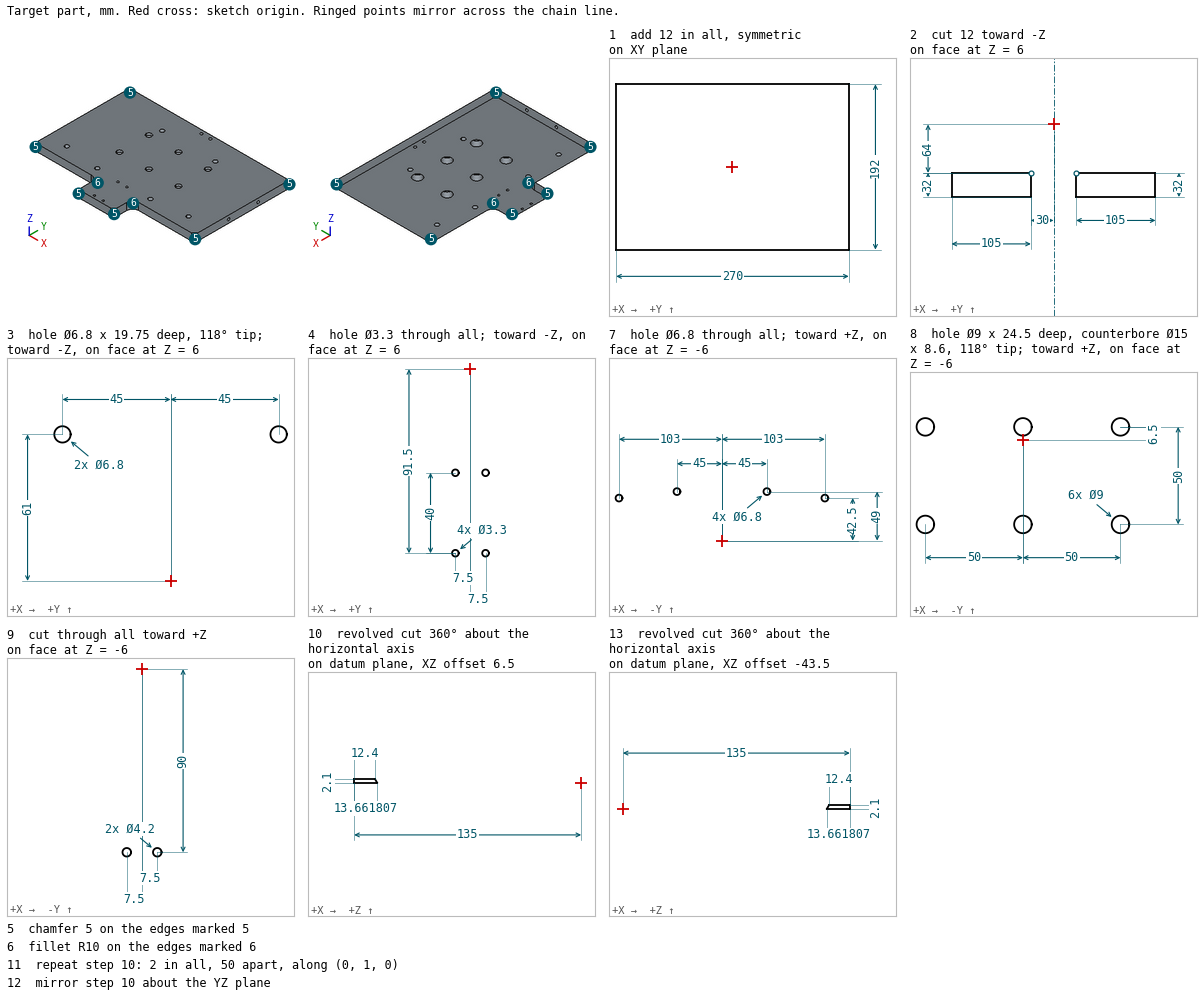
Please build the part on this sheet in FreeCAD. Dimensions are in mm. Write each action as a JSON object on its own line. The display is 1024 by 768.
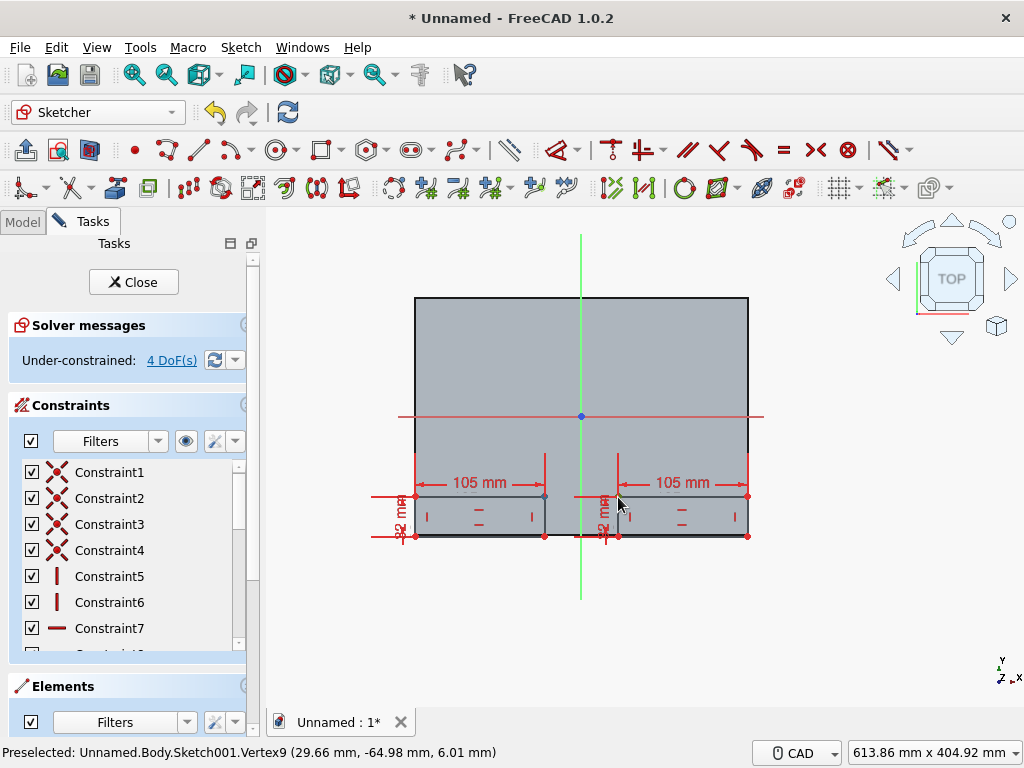
{"action": "left_click", "coordinate": [581, 584]}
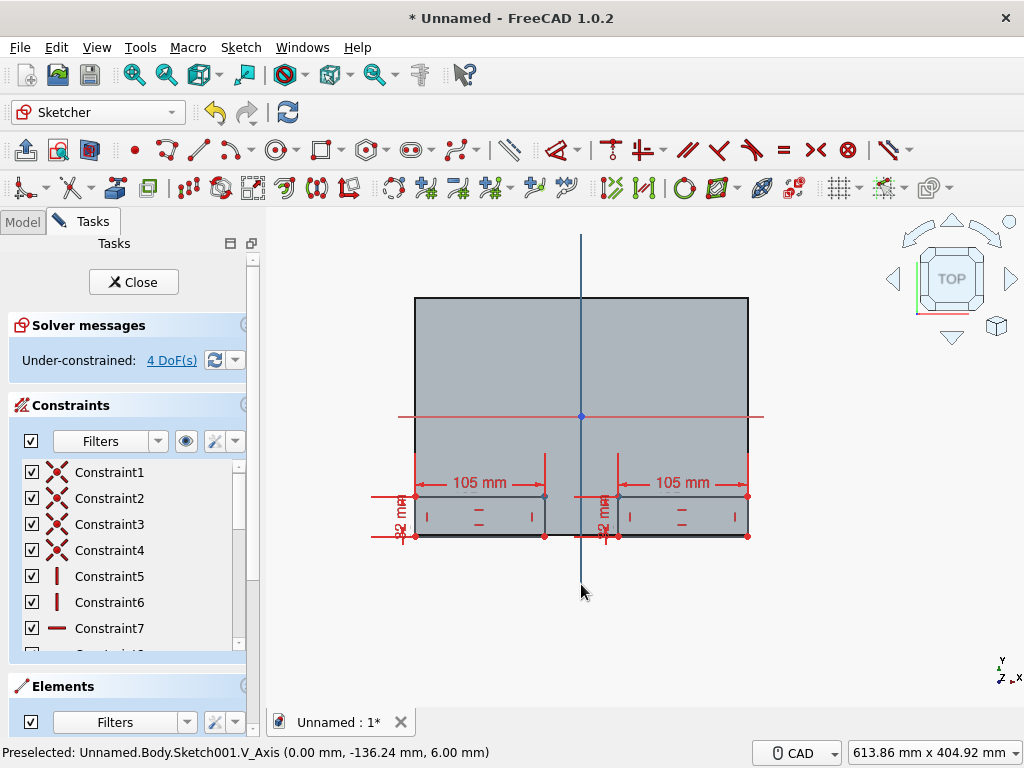
{"action": "key", "text": "s"}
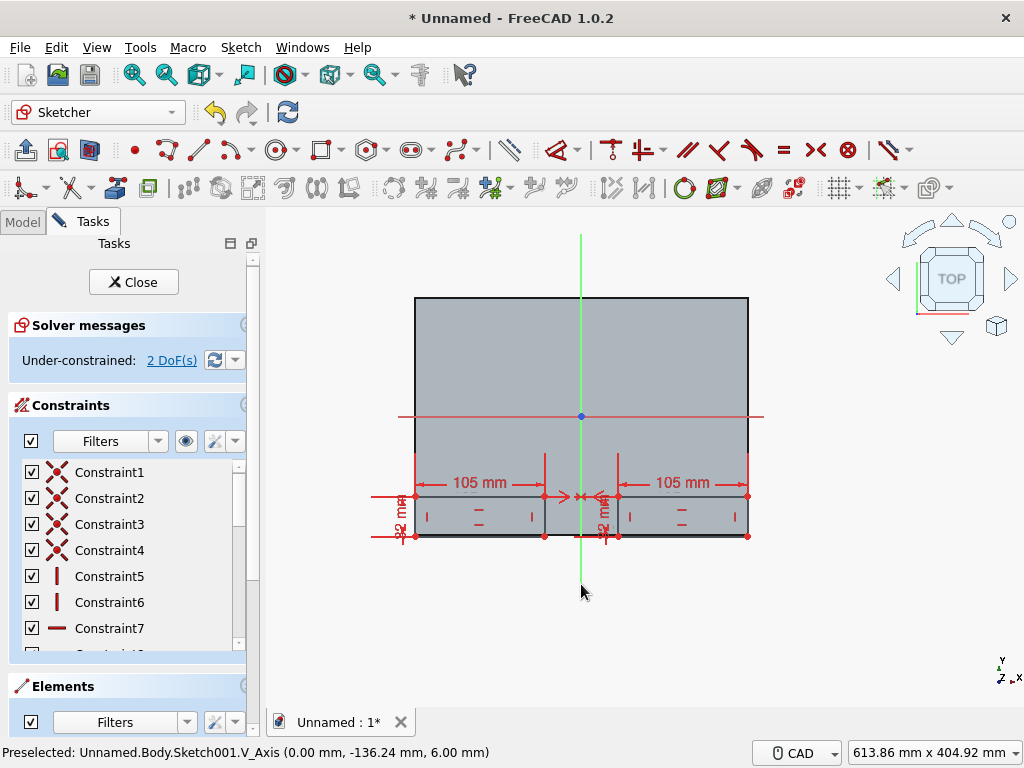
{"action": "key", "text": "d"}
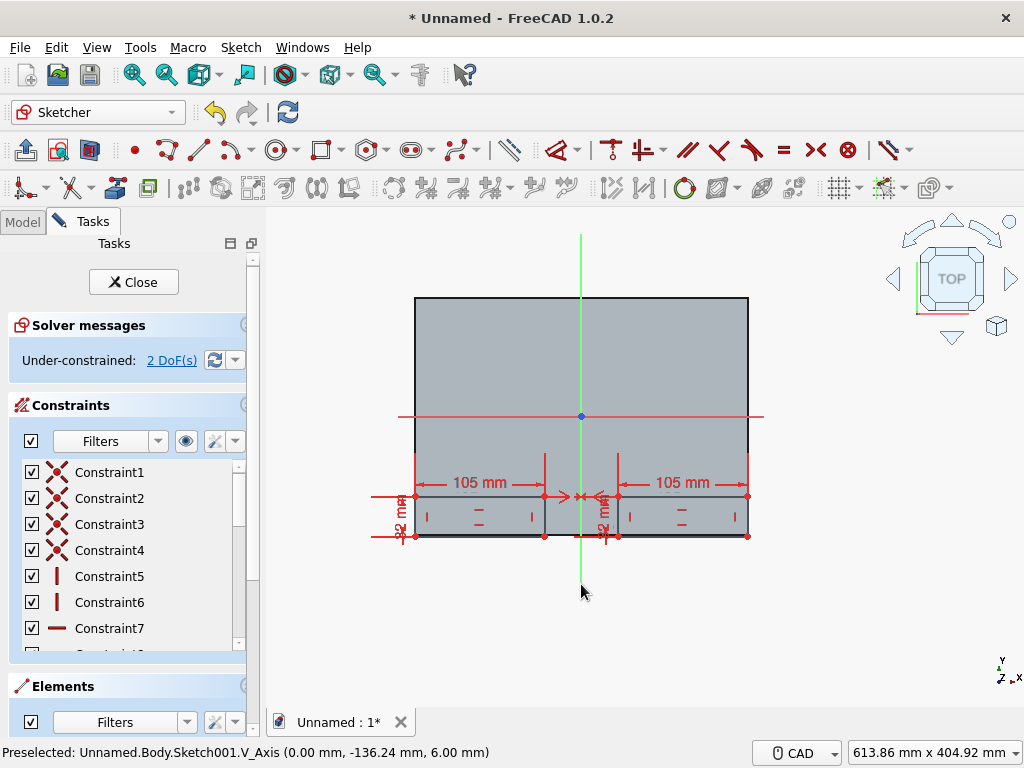
{"action": "left_click", "coordinate": [415, 497]}
{"action": "left_click", "coordinate": [381, 457]}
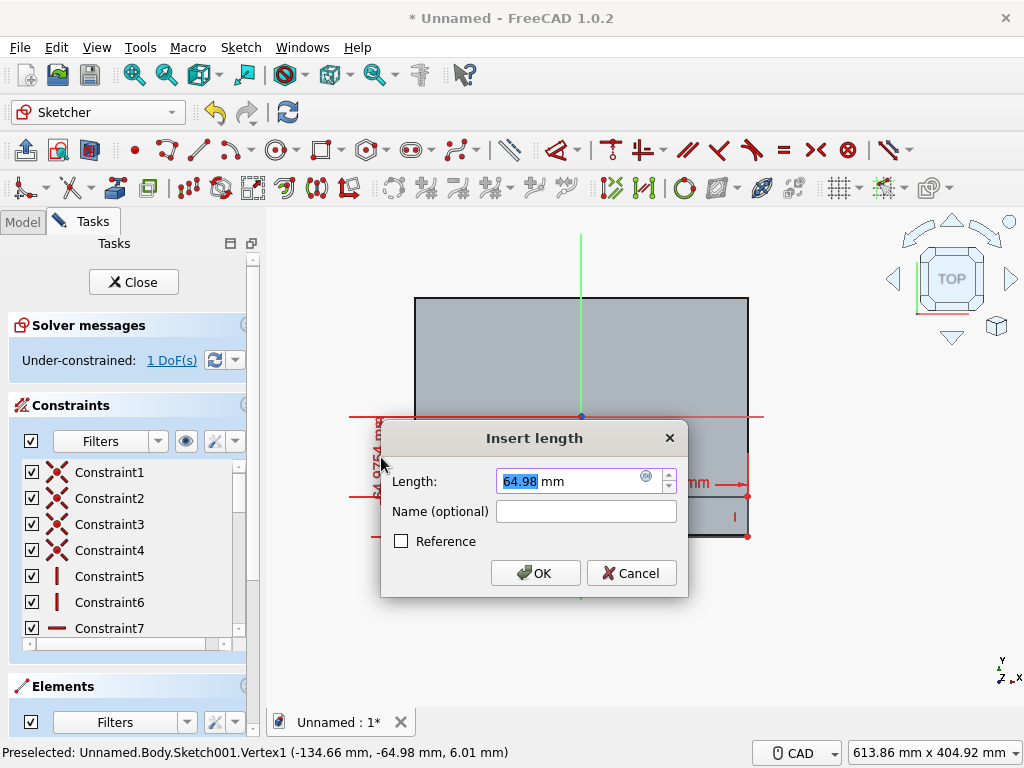
{"action": "type", "text": "64"}
{"action": "key", "text": "Return"}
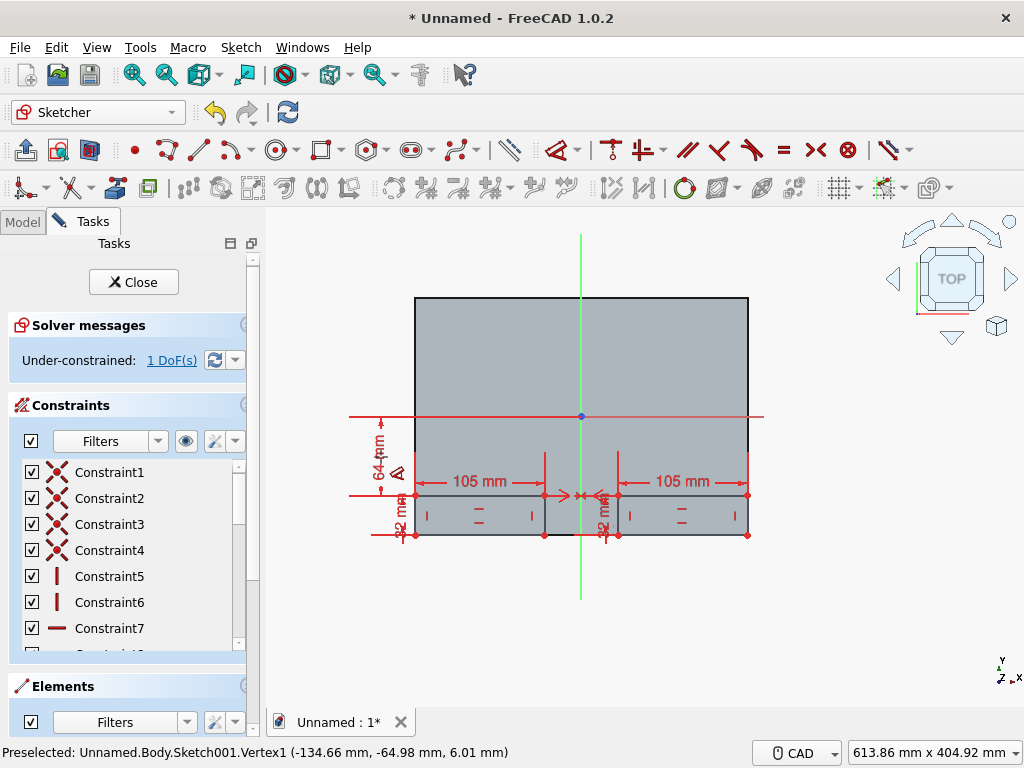
{"action": "left_click", "coordinate": [545, 535]}
{"action": "left_click", "coordinate": [563, 569]}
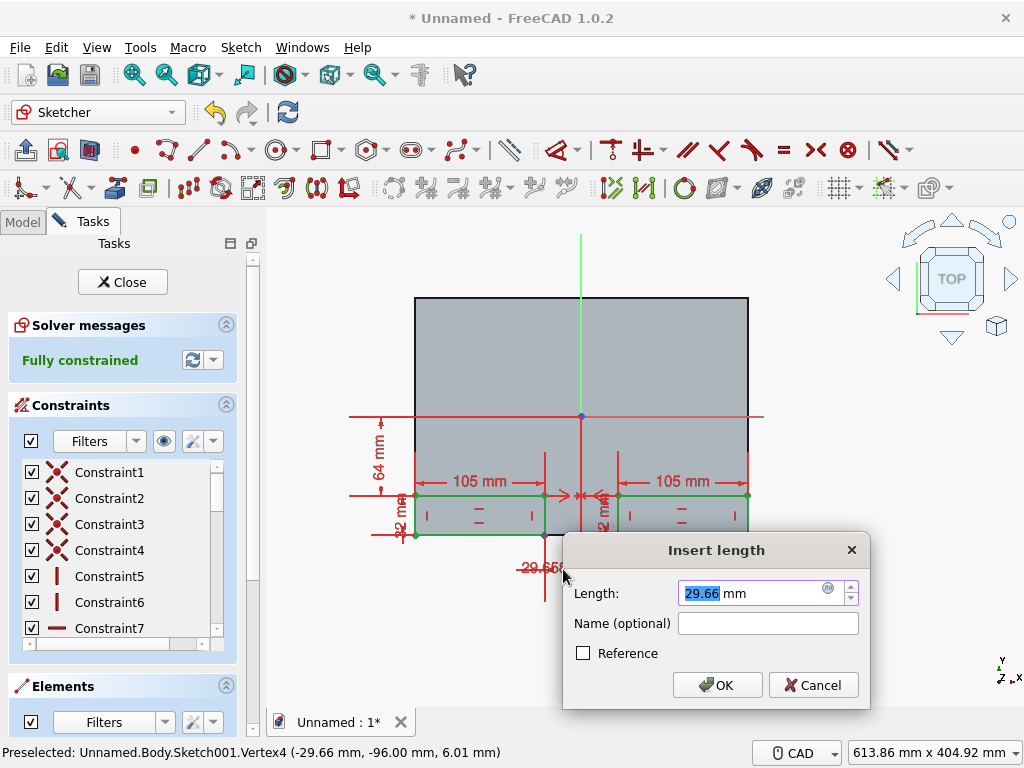
{"action": "type", "text": "30"}
{"action": "key", "text": "Return"}
{"action": "key", "text": "Escape"}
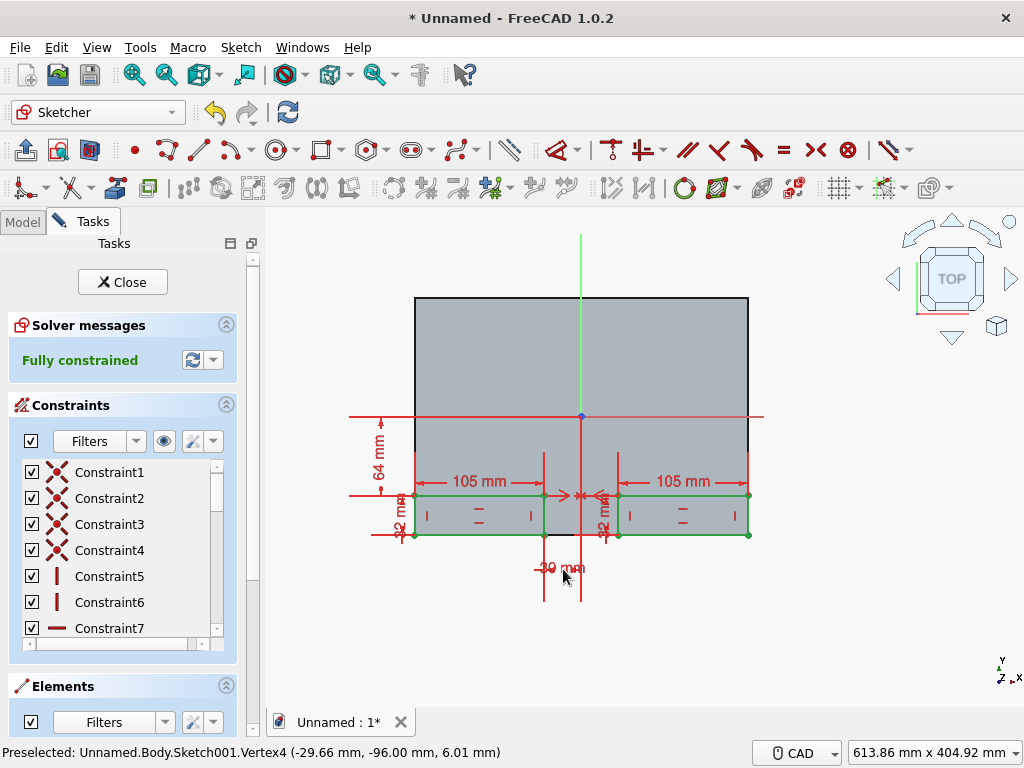
{"action": "left_click", "coordinate": [123, 282]}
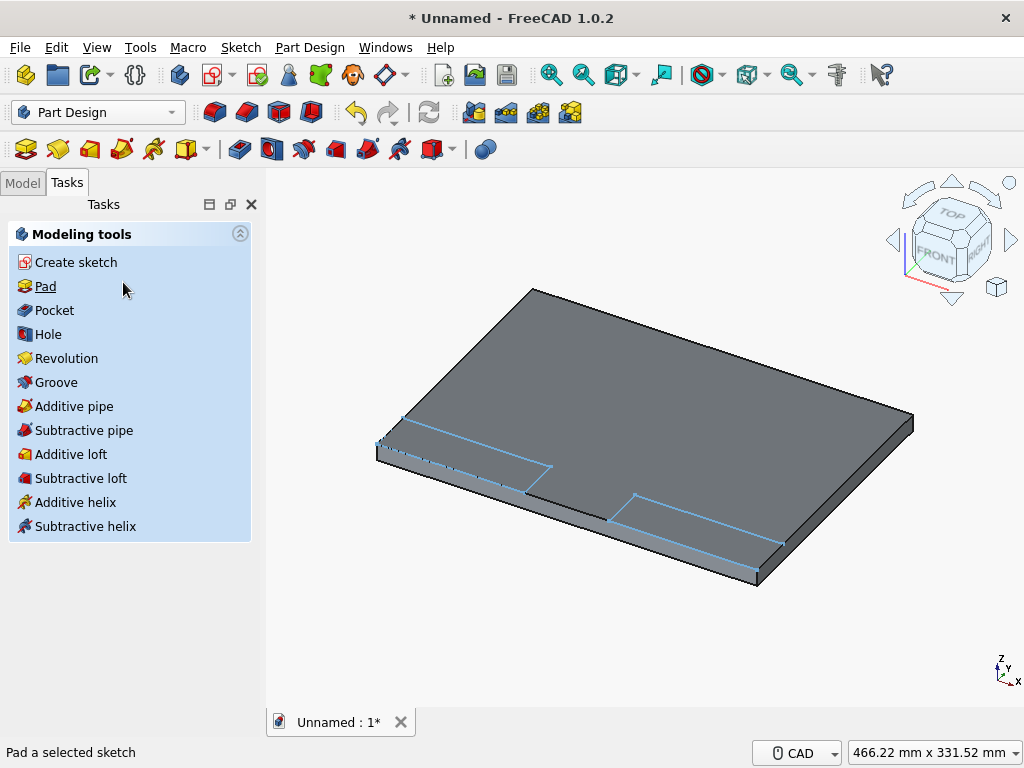
{"action": "left_click", "coordinate": [240, 150]}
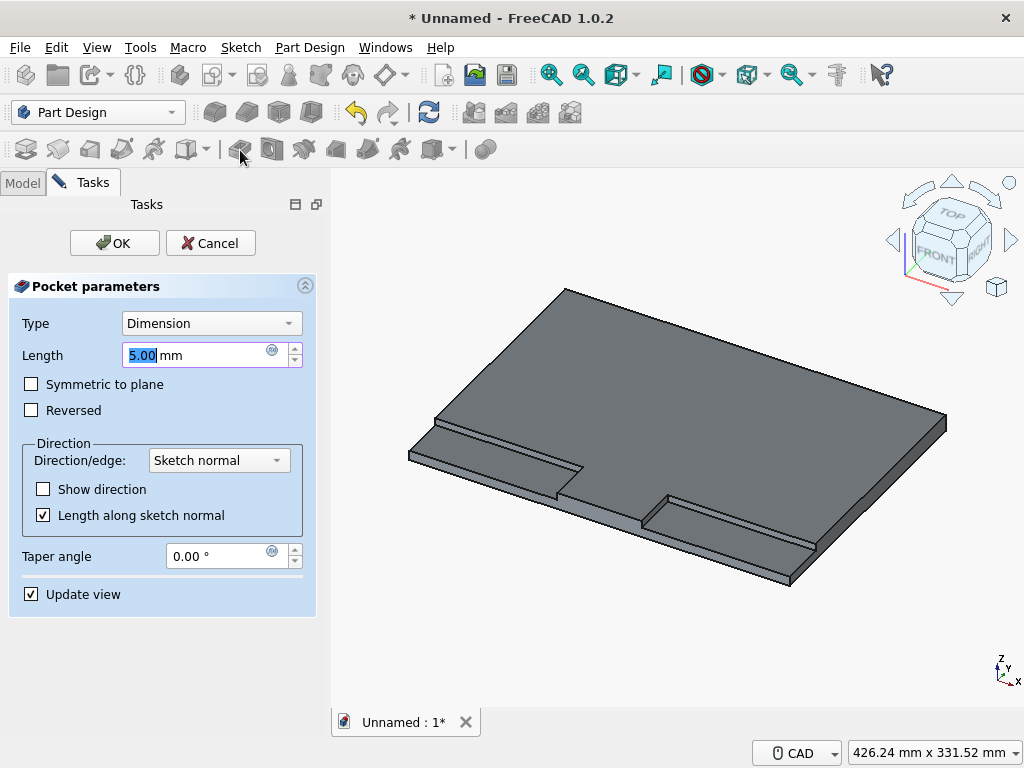
{"action": "type", "text": "12"}
{"action": "key", "text": "Tab"}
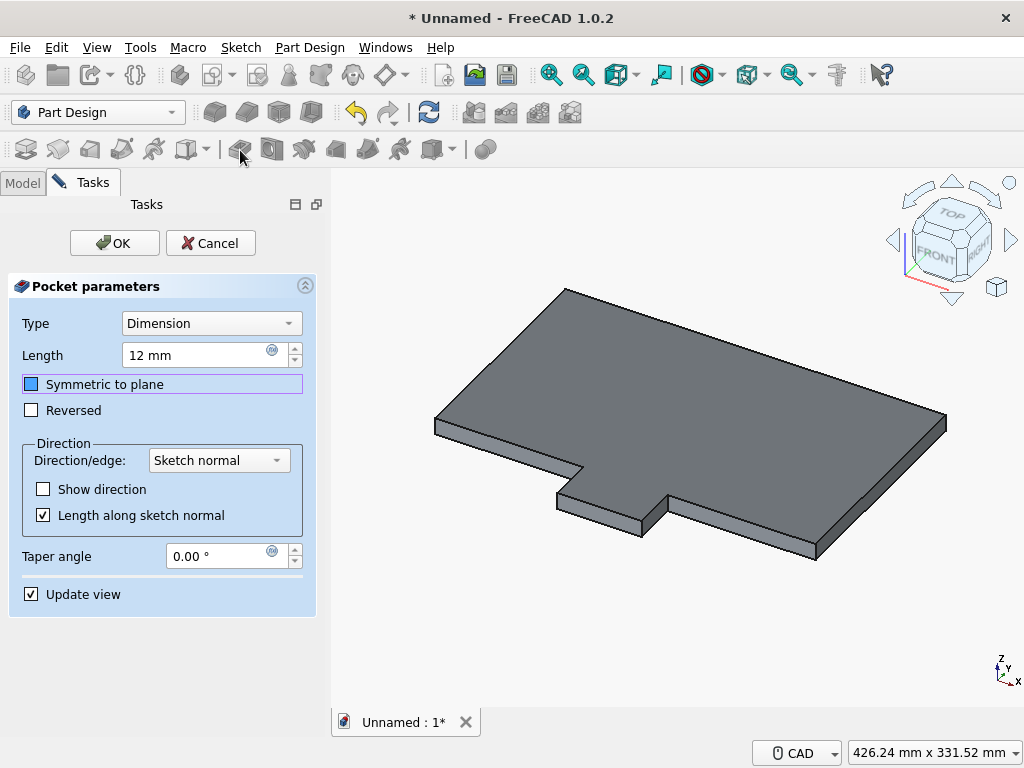
{"action": "left_click", "coordinate": [115, 243]}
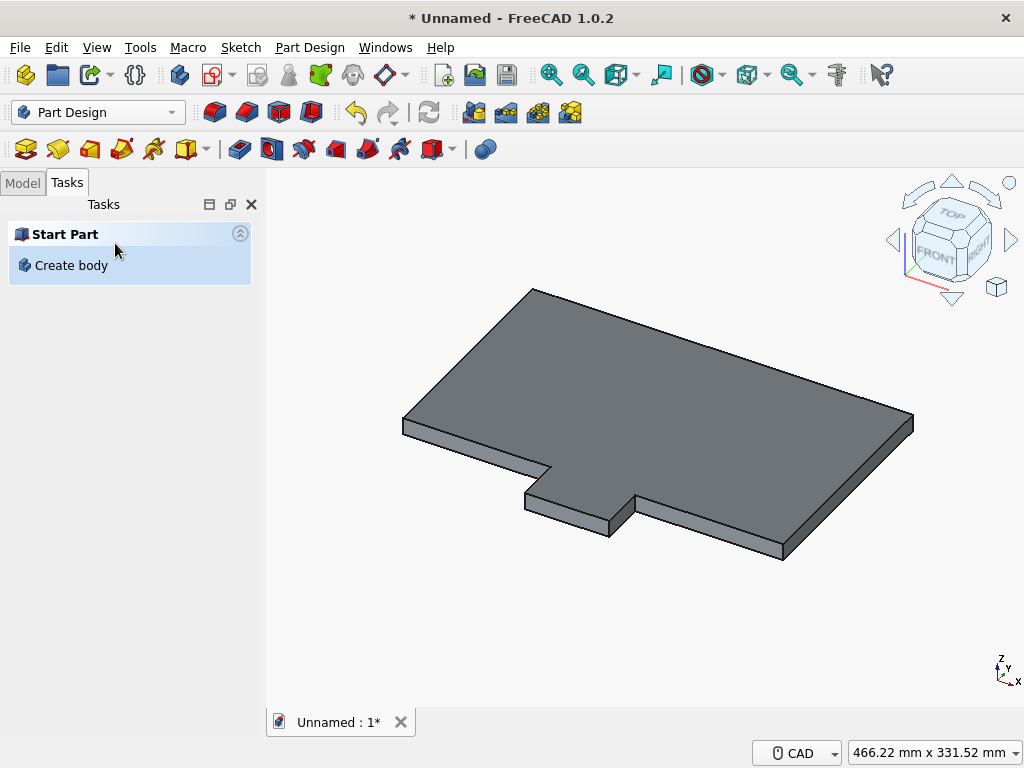
{"action": "left_click", "coordinate": [645, 429]}